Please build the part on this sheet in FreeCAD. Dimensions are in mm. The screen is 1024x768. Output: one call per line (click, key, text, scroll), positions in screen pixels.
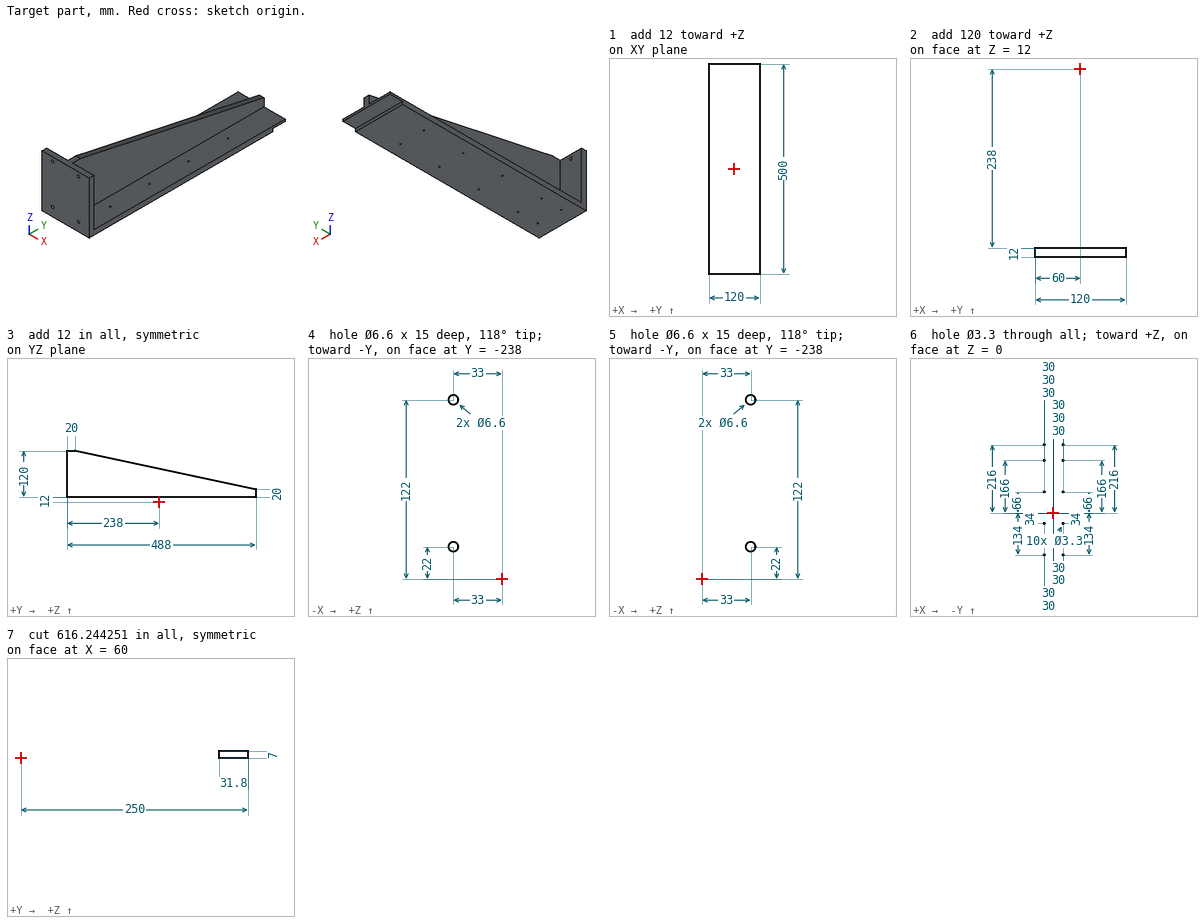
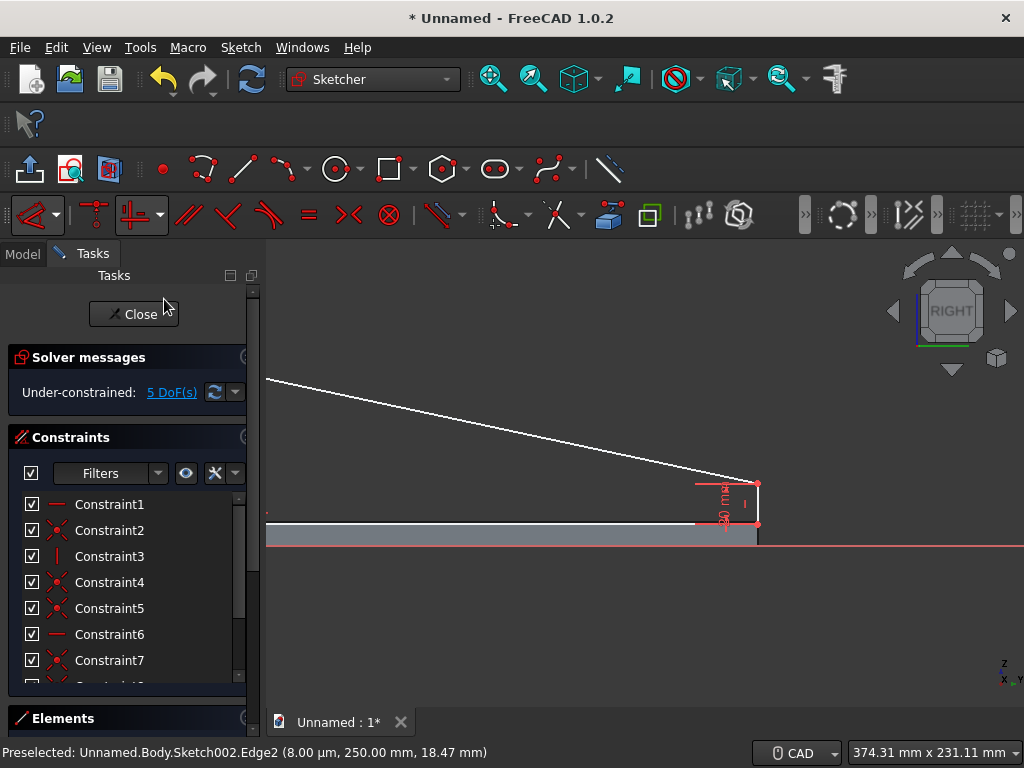
scroll(759, 508, down, 5)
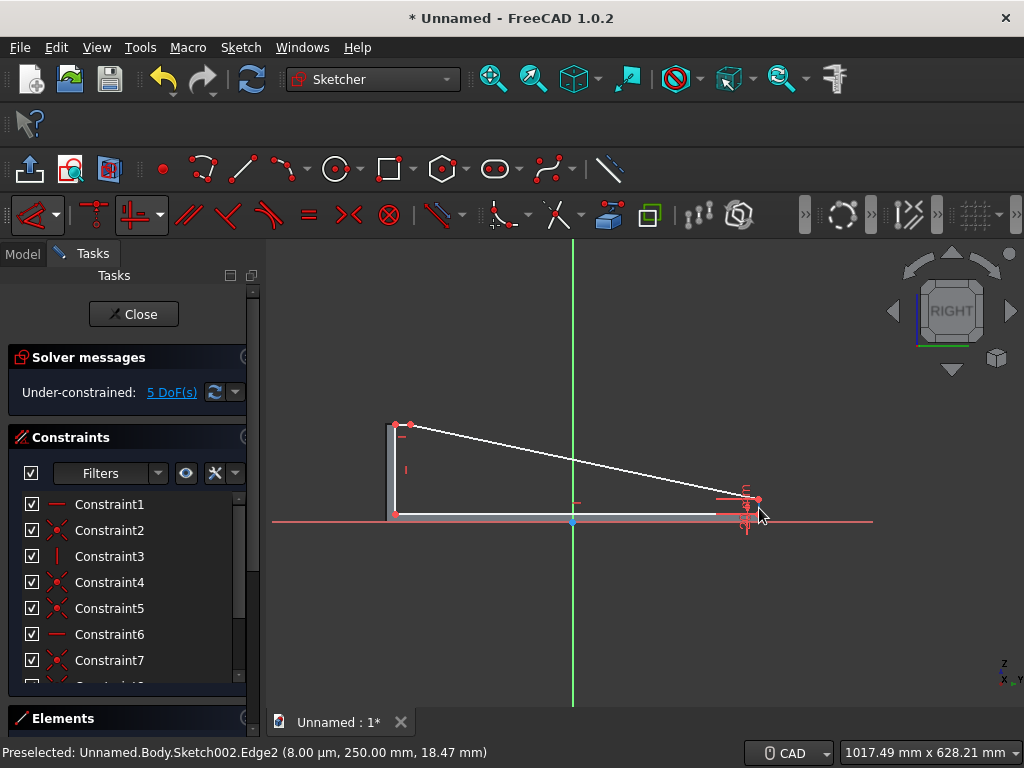
scroll(406, 425, up, 6)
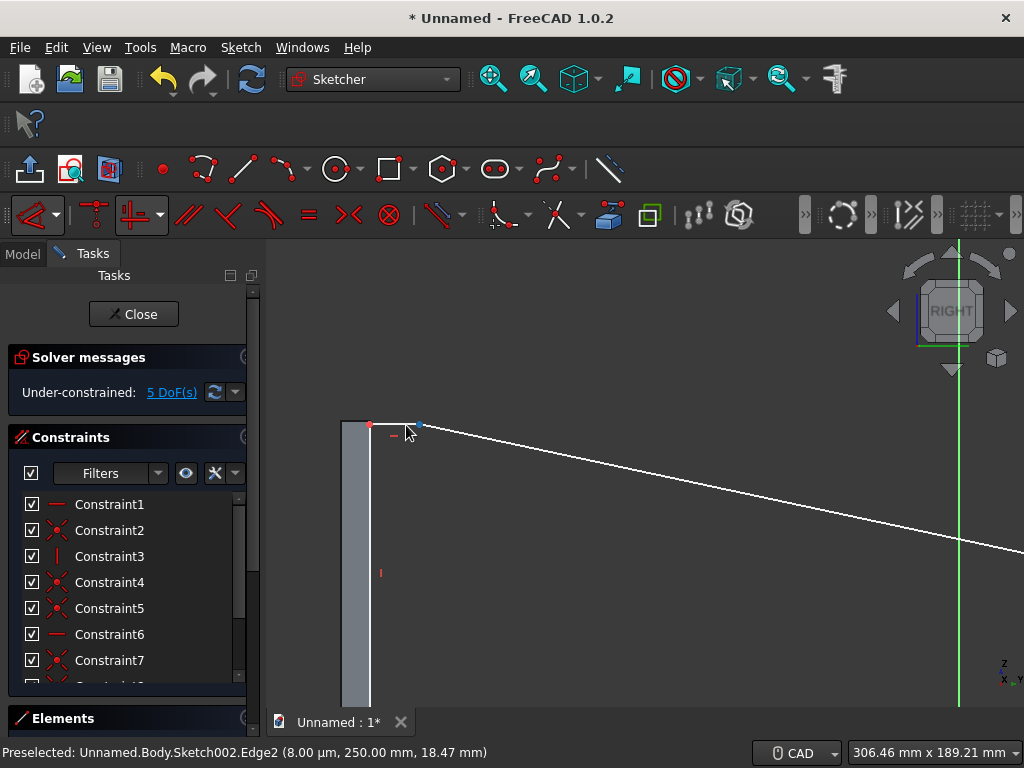
click(405, 424)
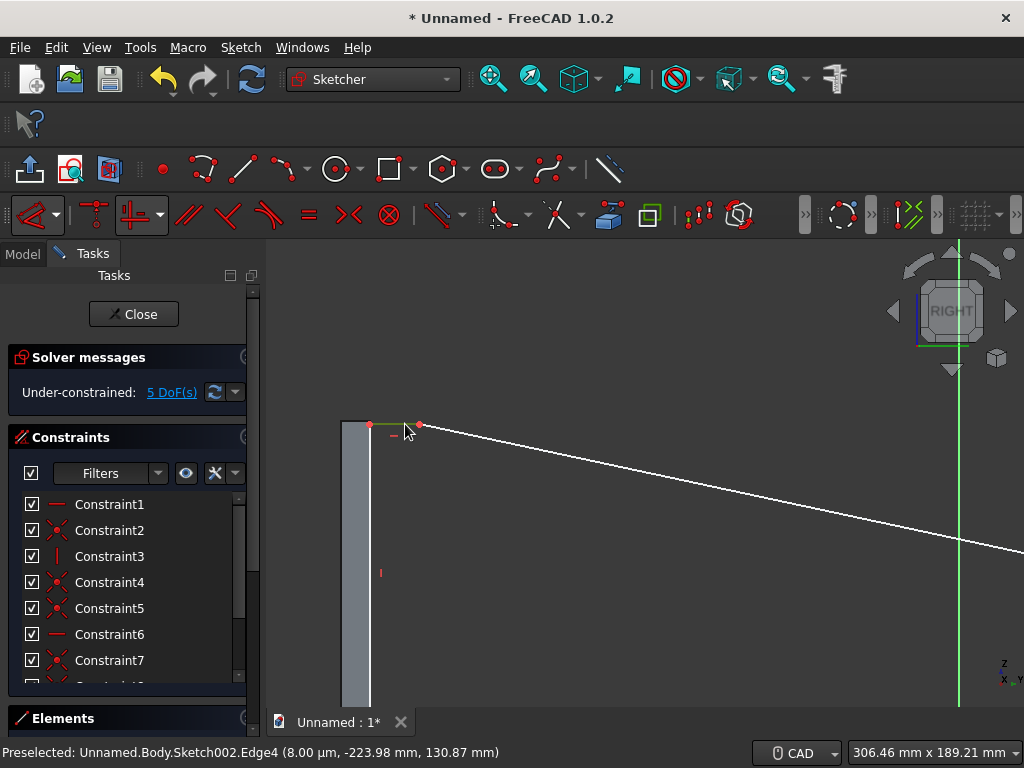
click(58, 216)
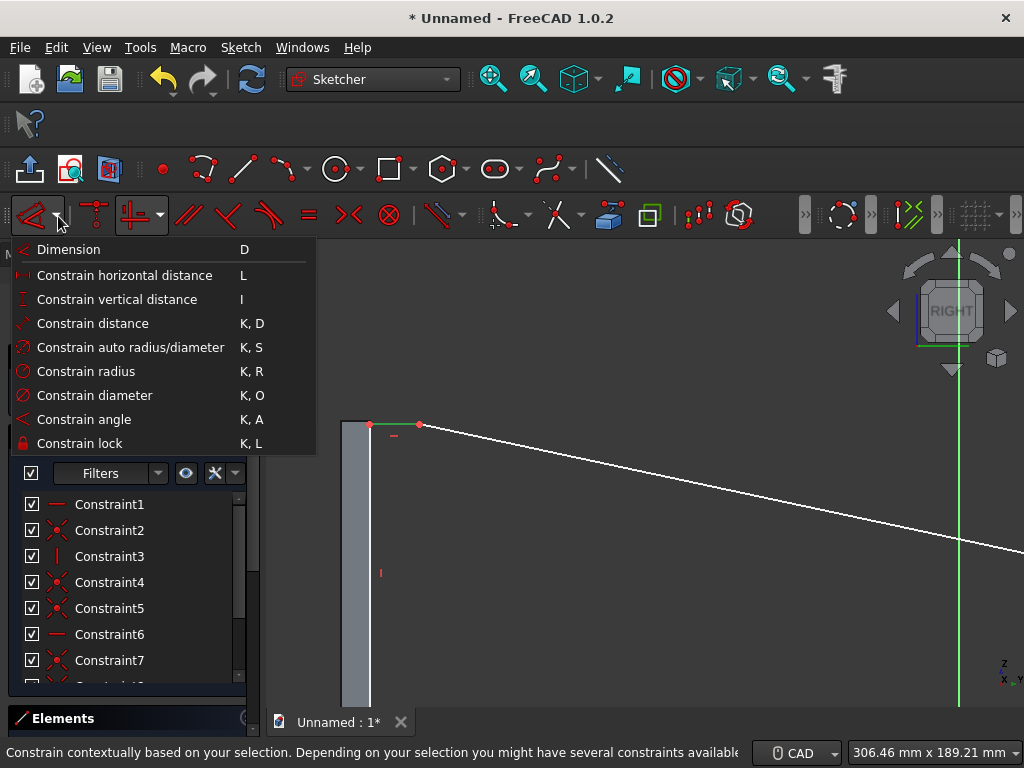
click(164, 275)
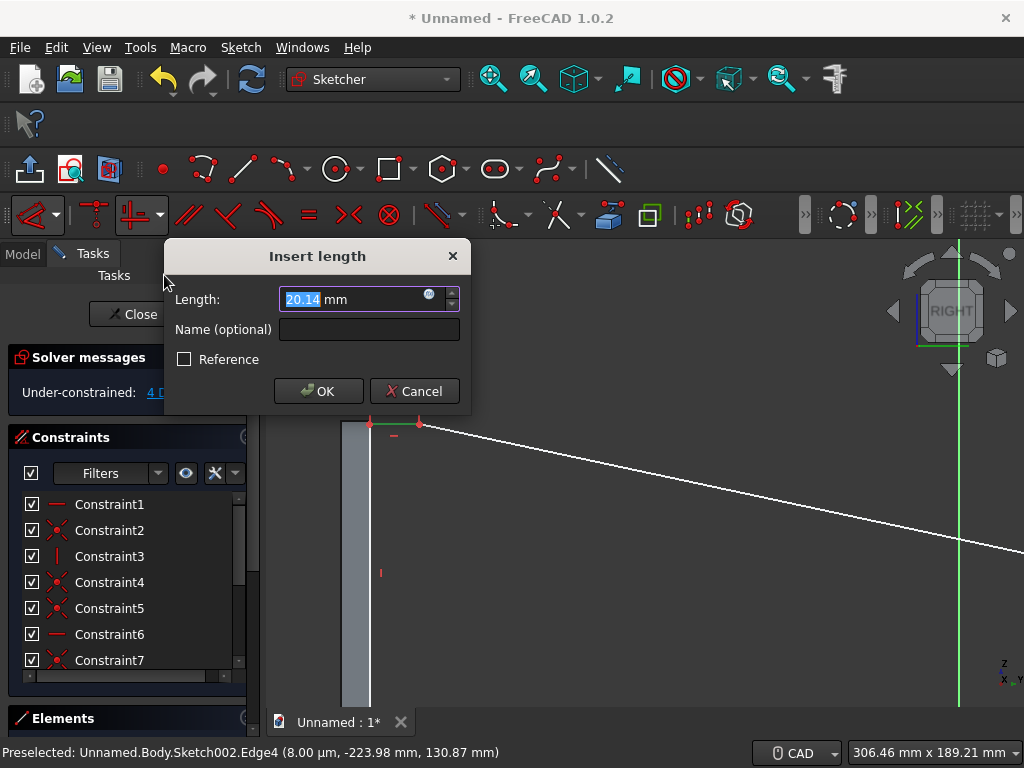
text(20)
key(Return)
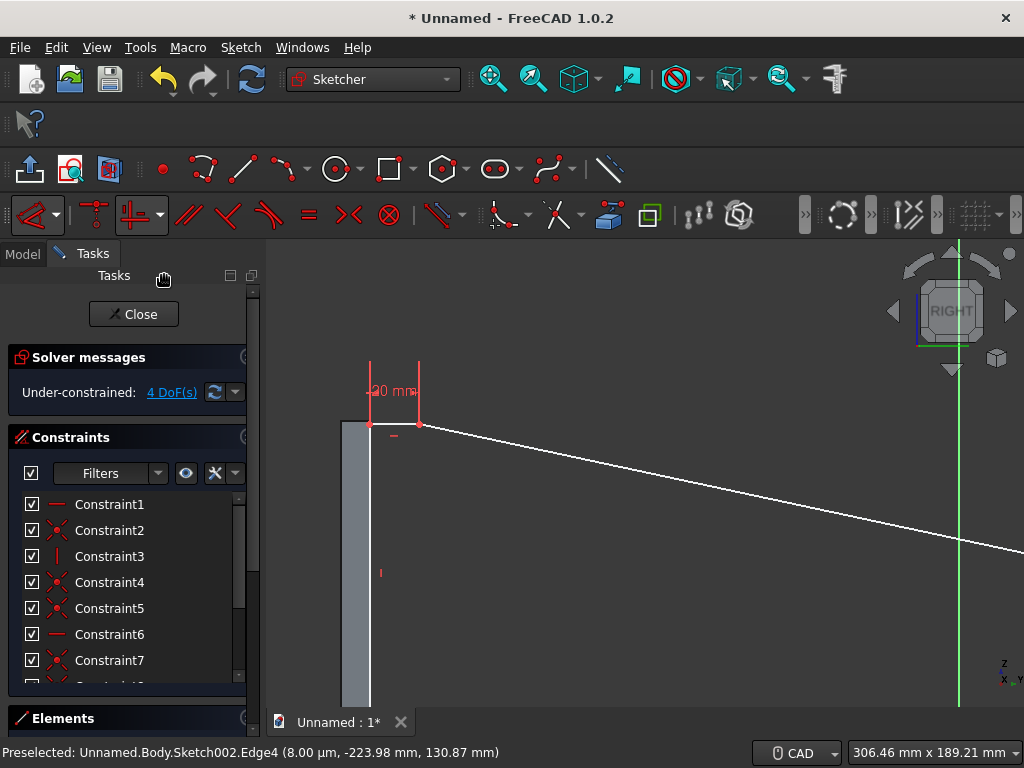
scroll(405, 425, down, 6)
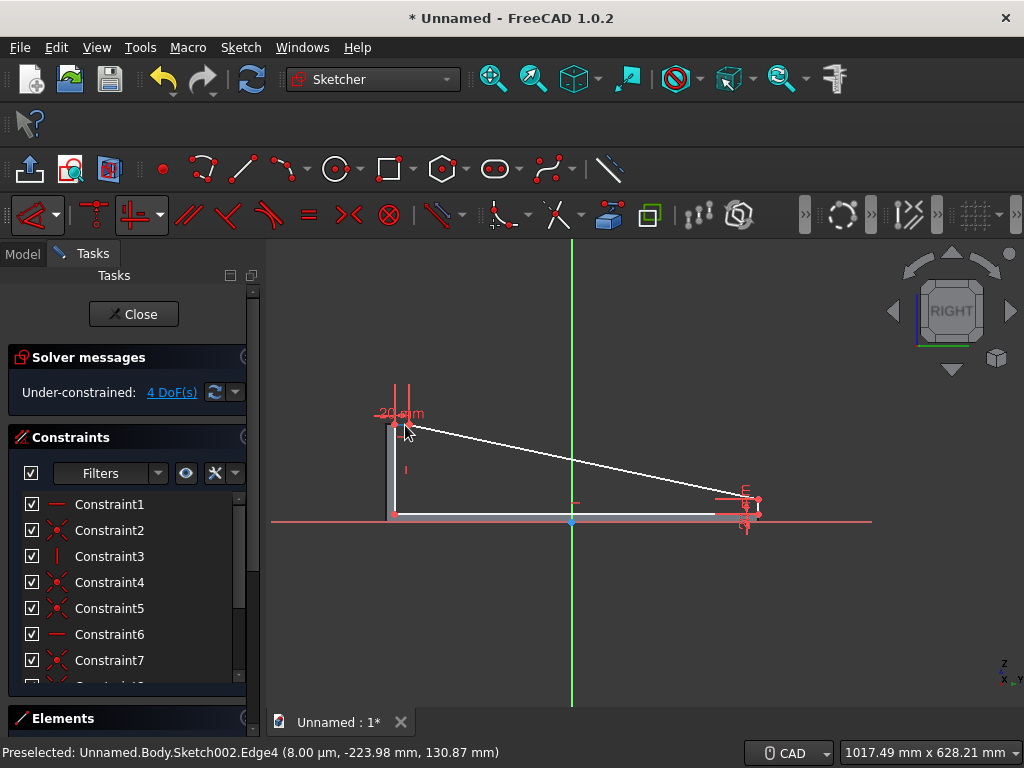
scroll(504, 514, up, 3)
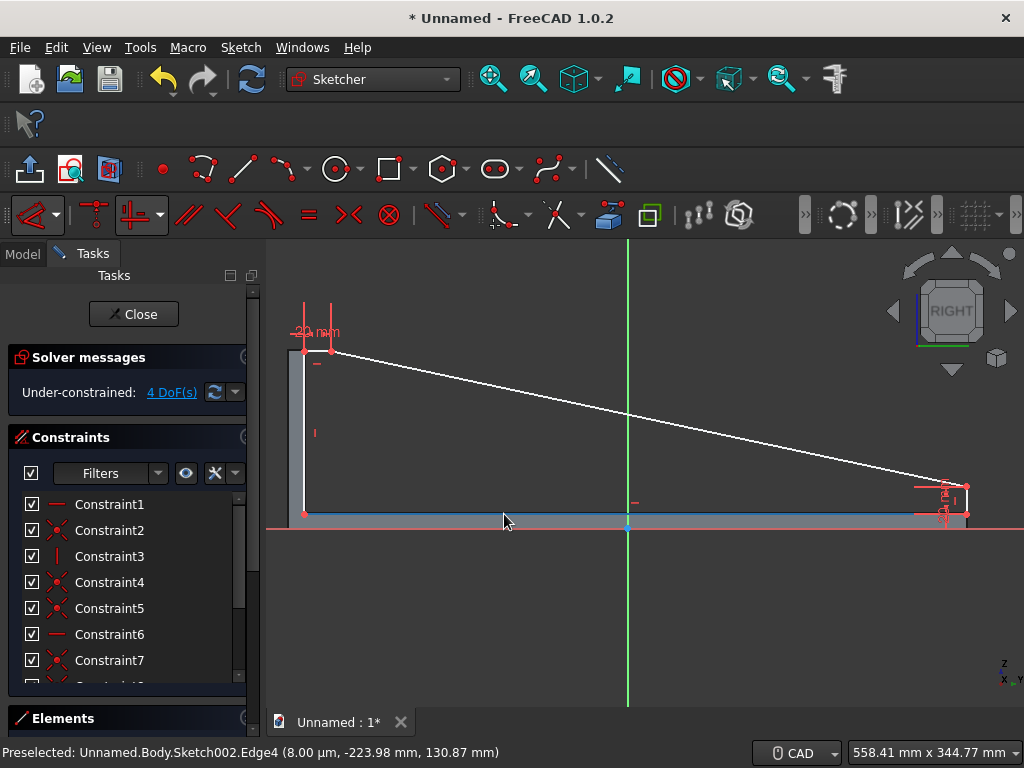
click(503, 514)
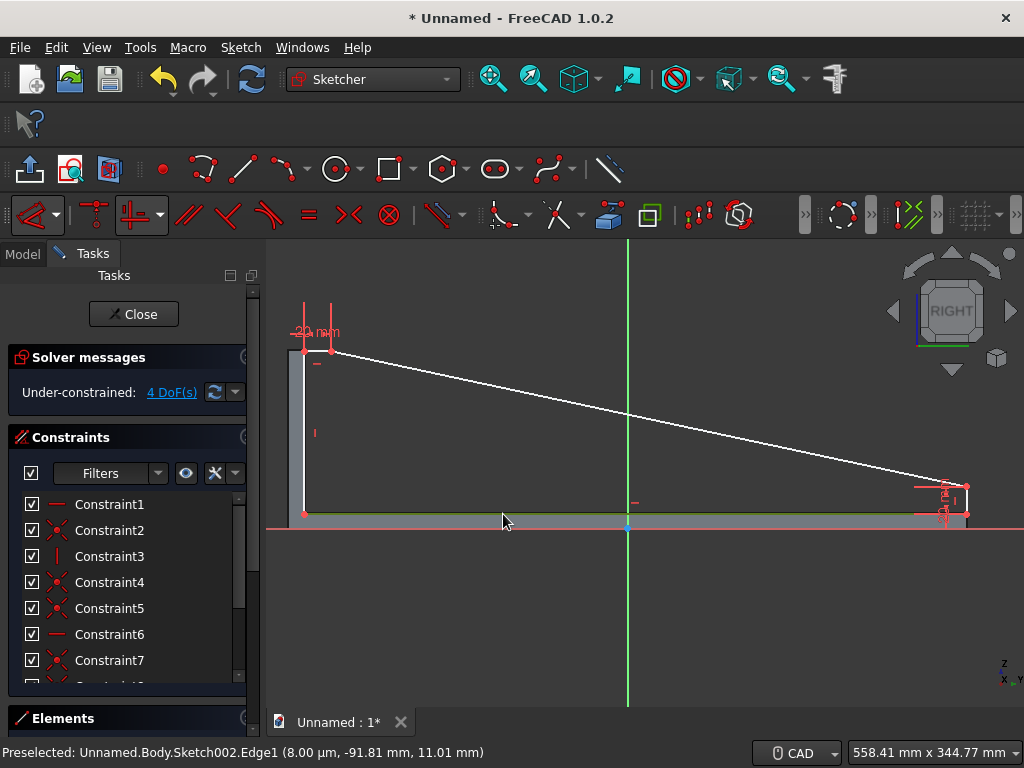
click(58, 216)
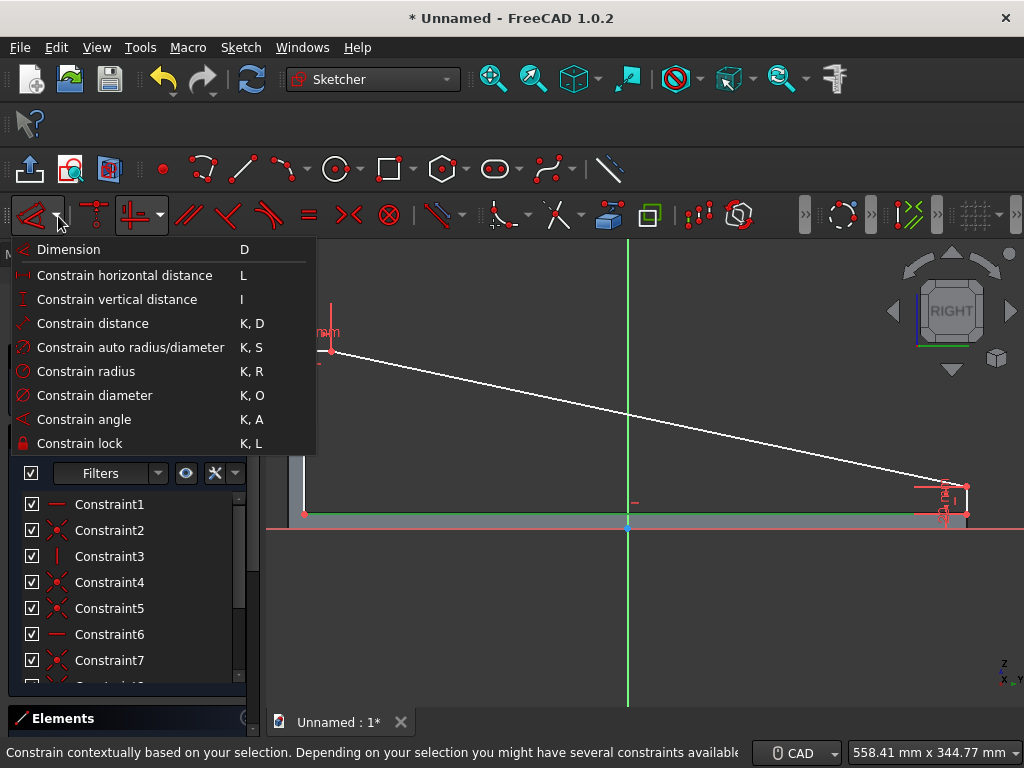
click(164, 275)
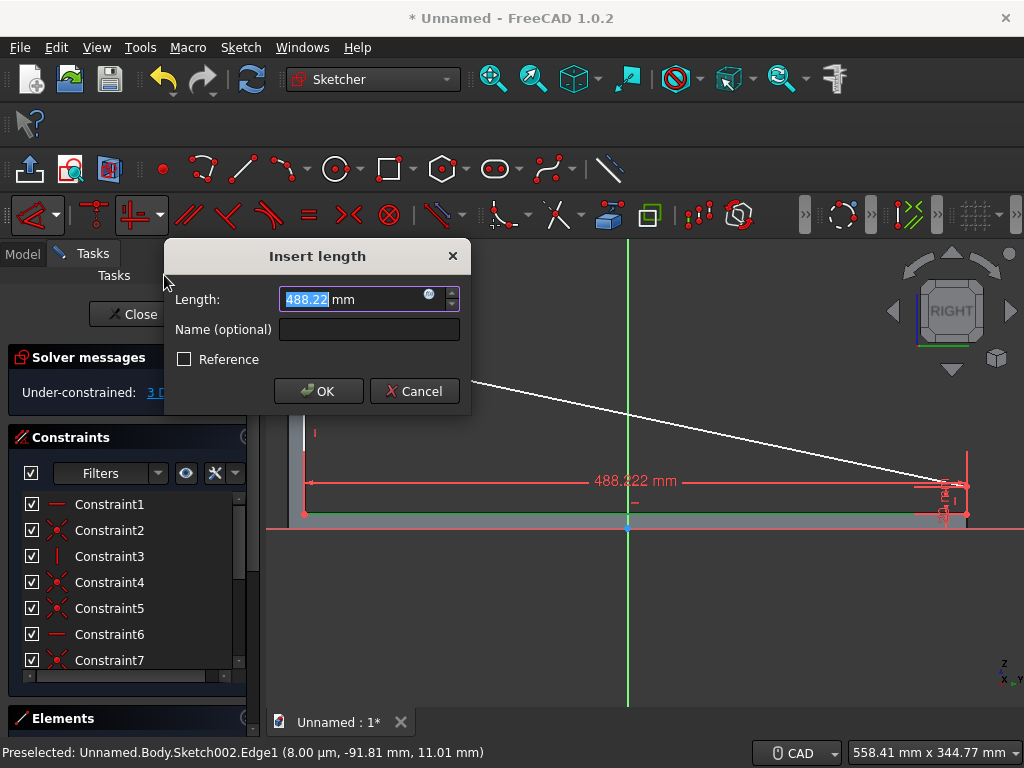
text(488)
key(Return)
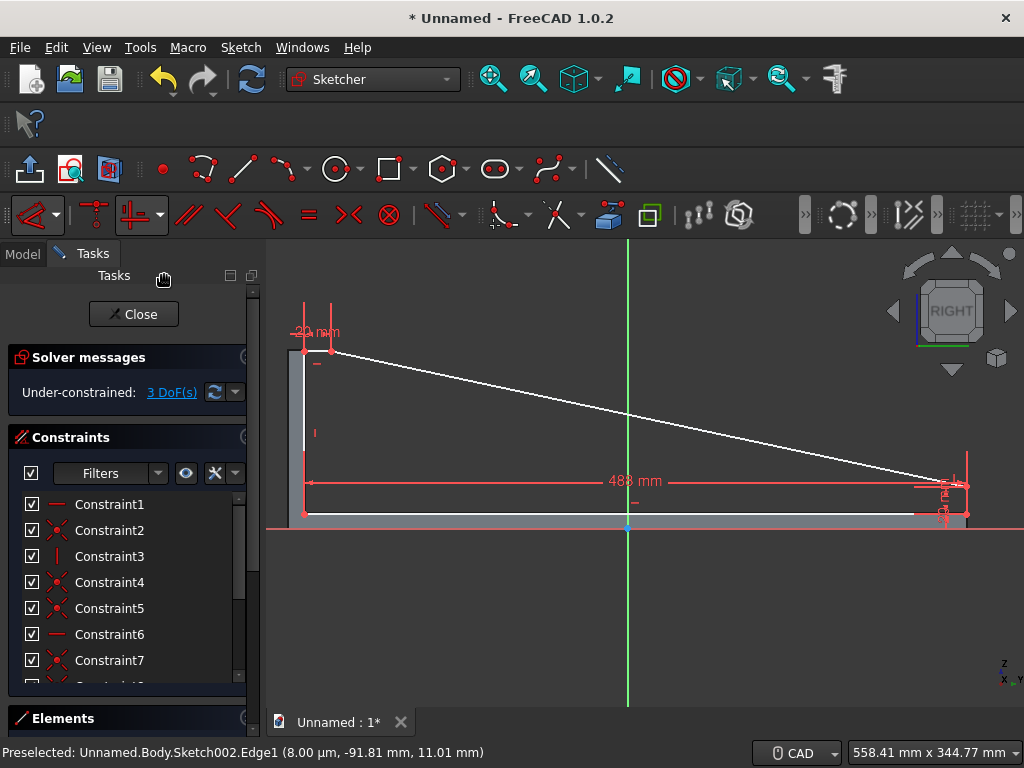
click(304, 400)